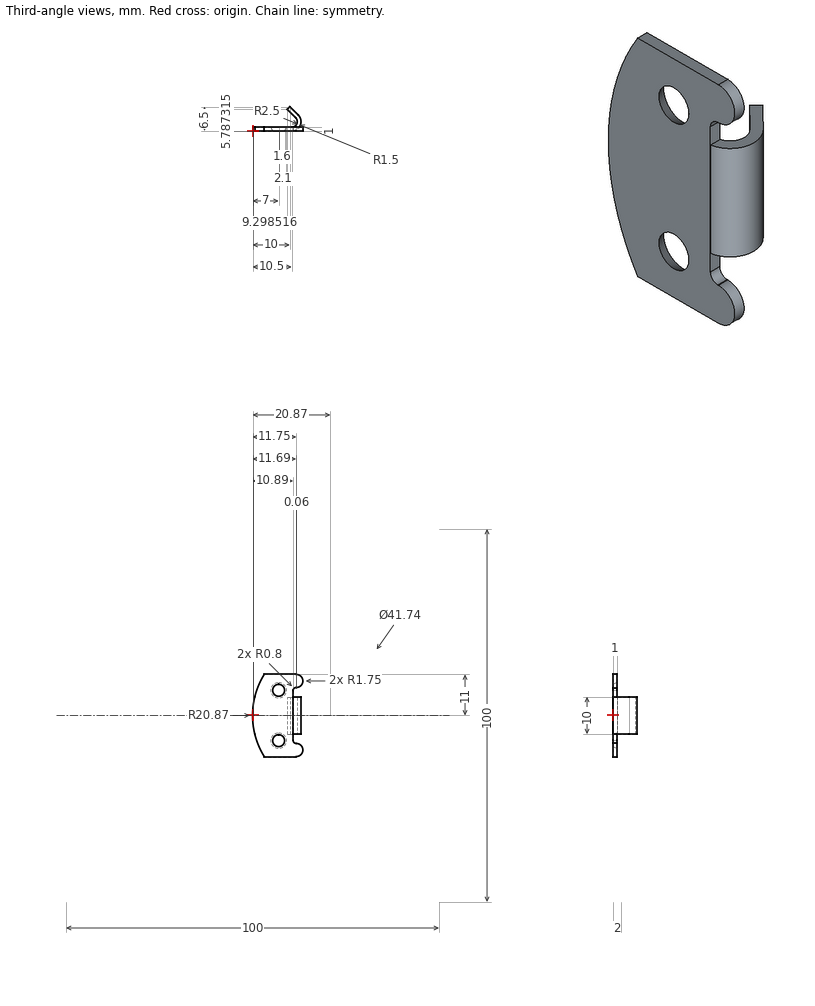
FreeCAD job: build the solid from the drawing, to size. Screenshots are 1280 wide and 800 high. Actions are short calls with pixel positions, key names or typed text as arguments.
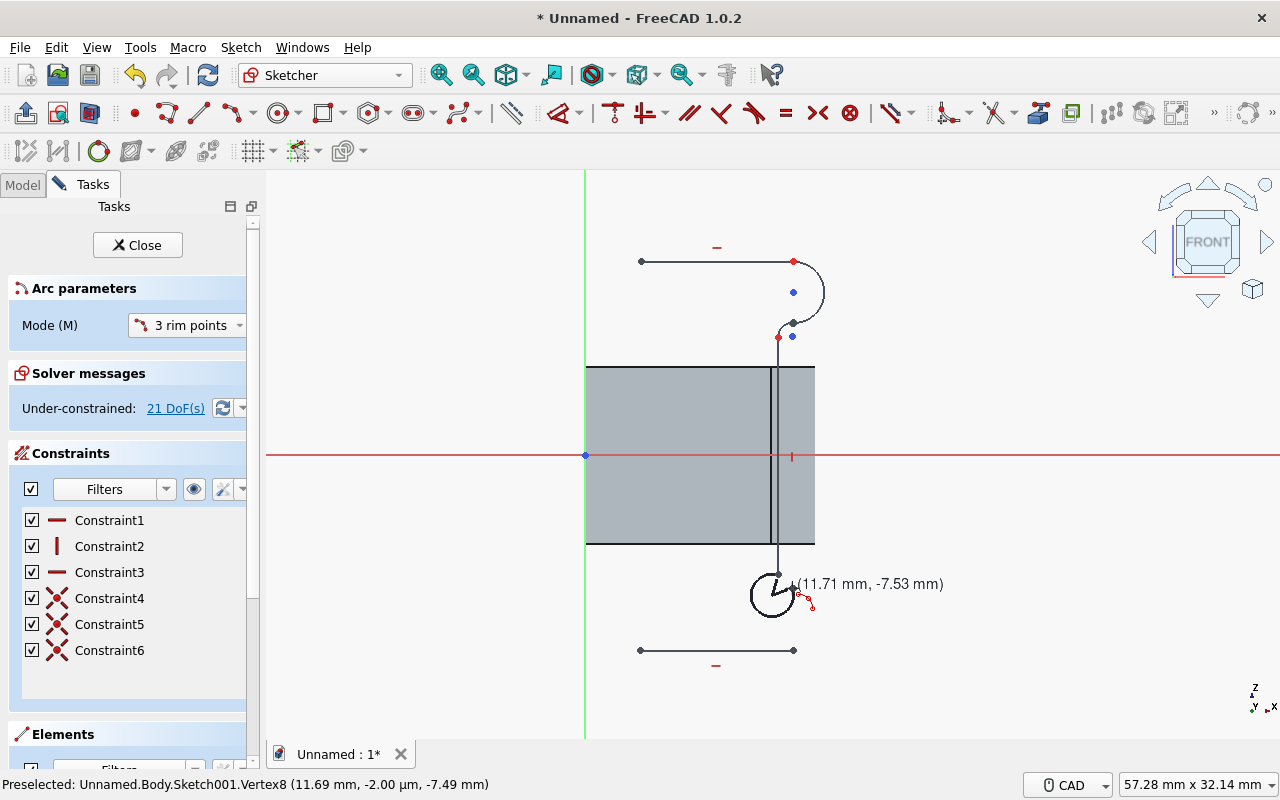
scroll(782, 584, up, 7)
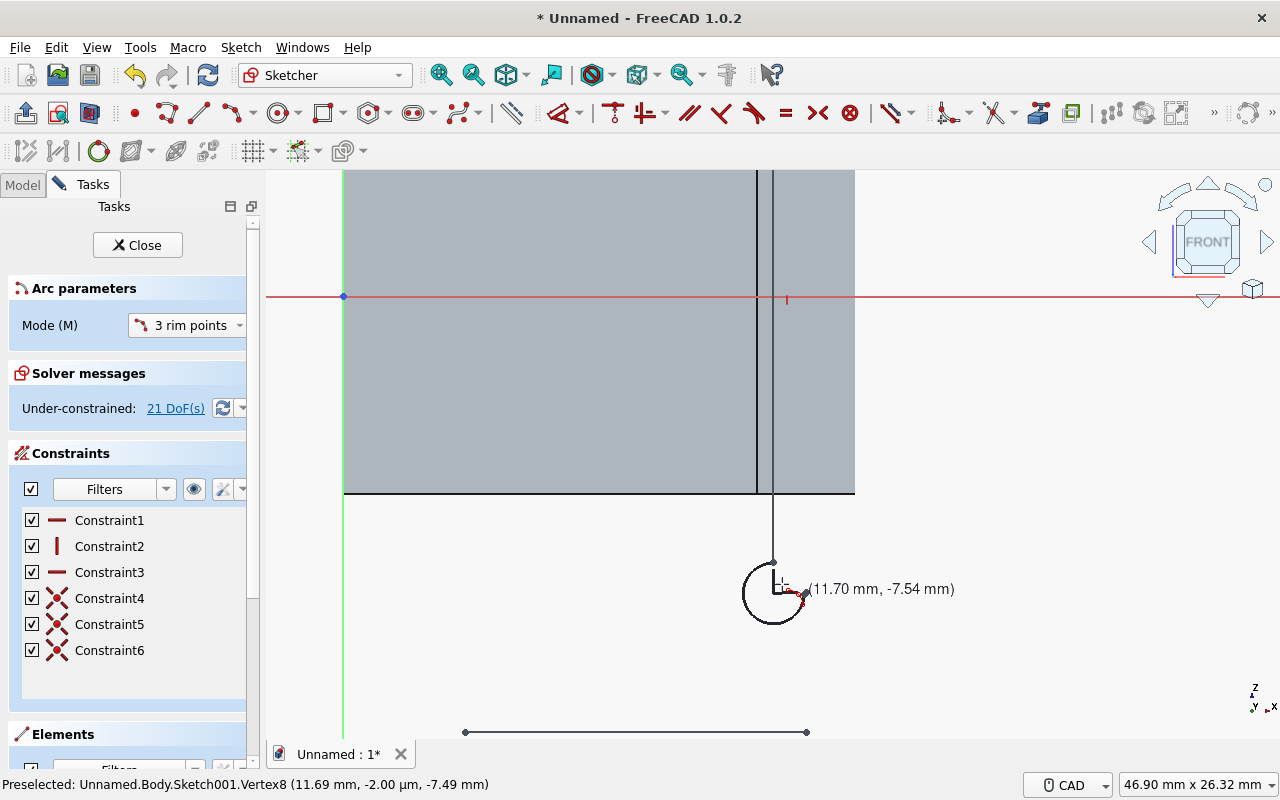
click(781, 582)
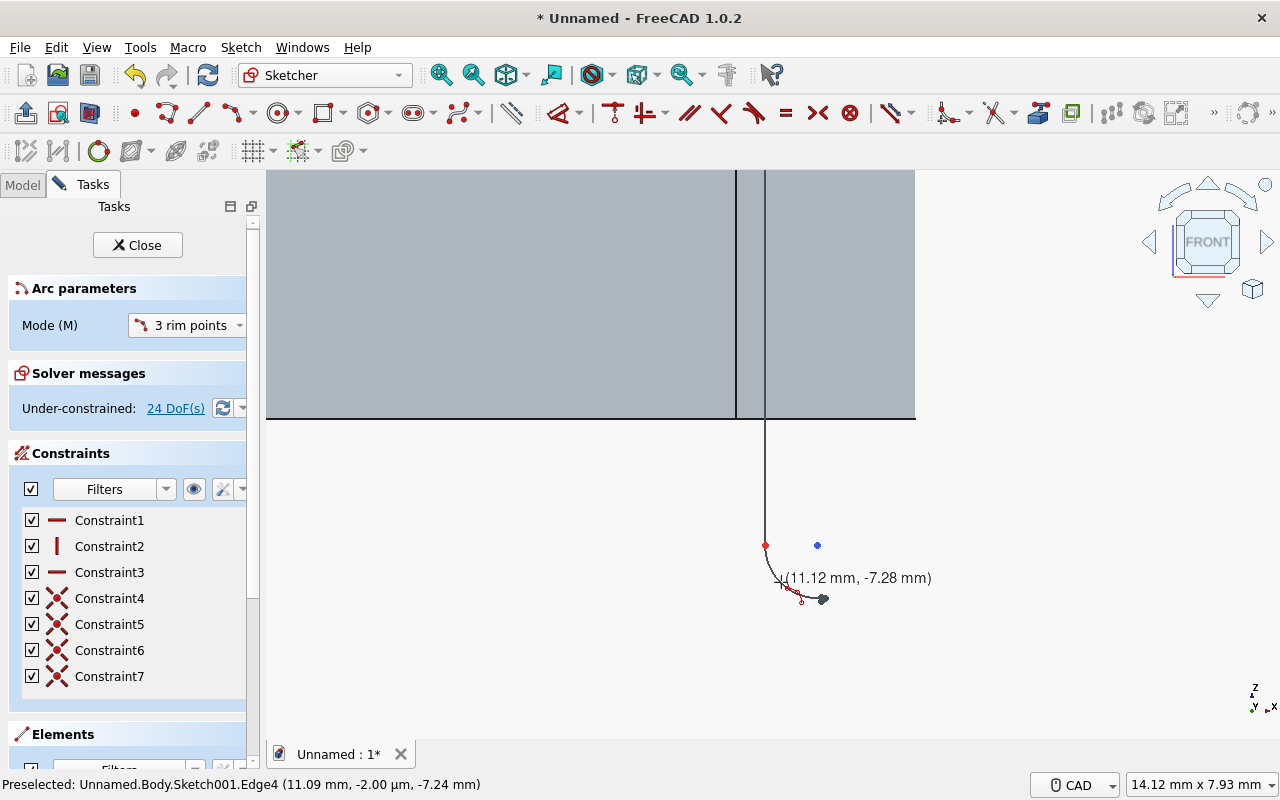
scroll(826, 599, up, 10)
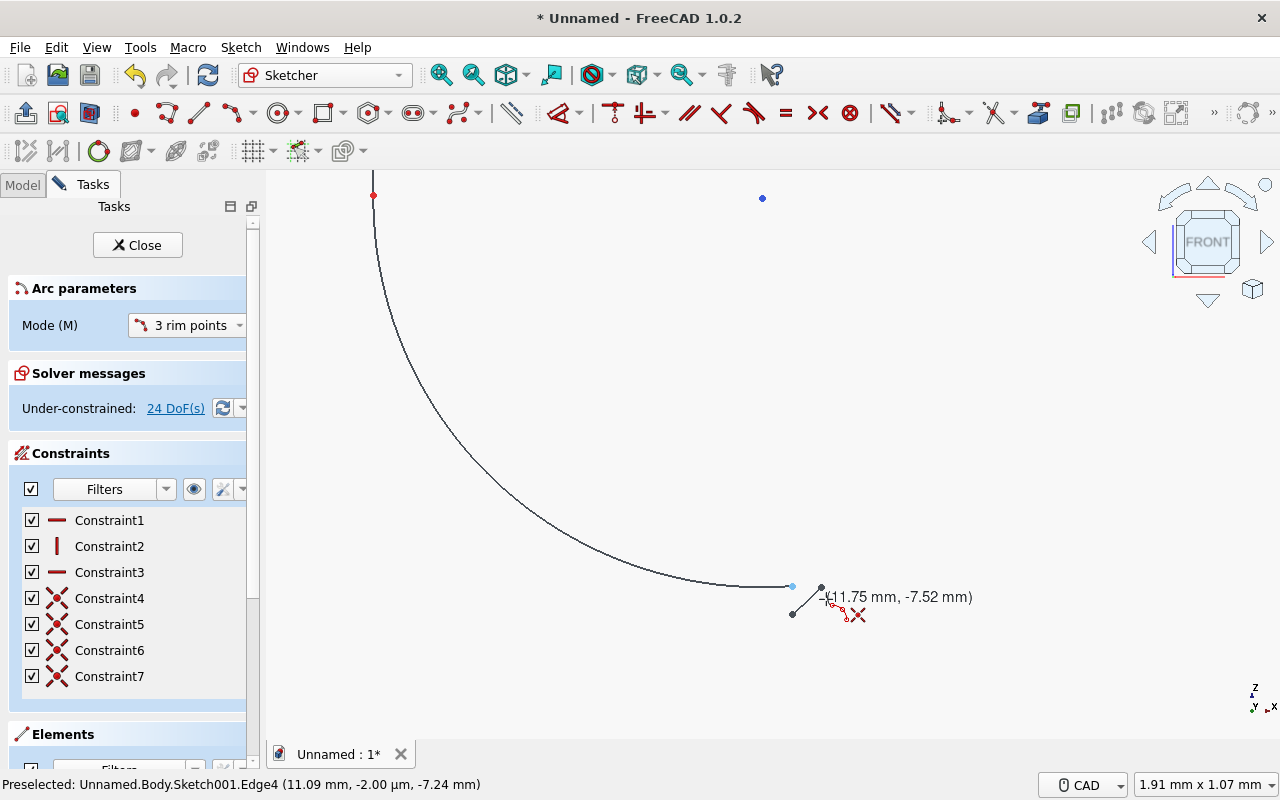
click(821, 587)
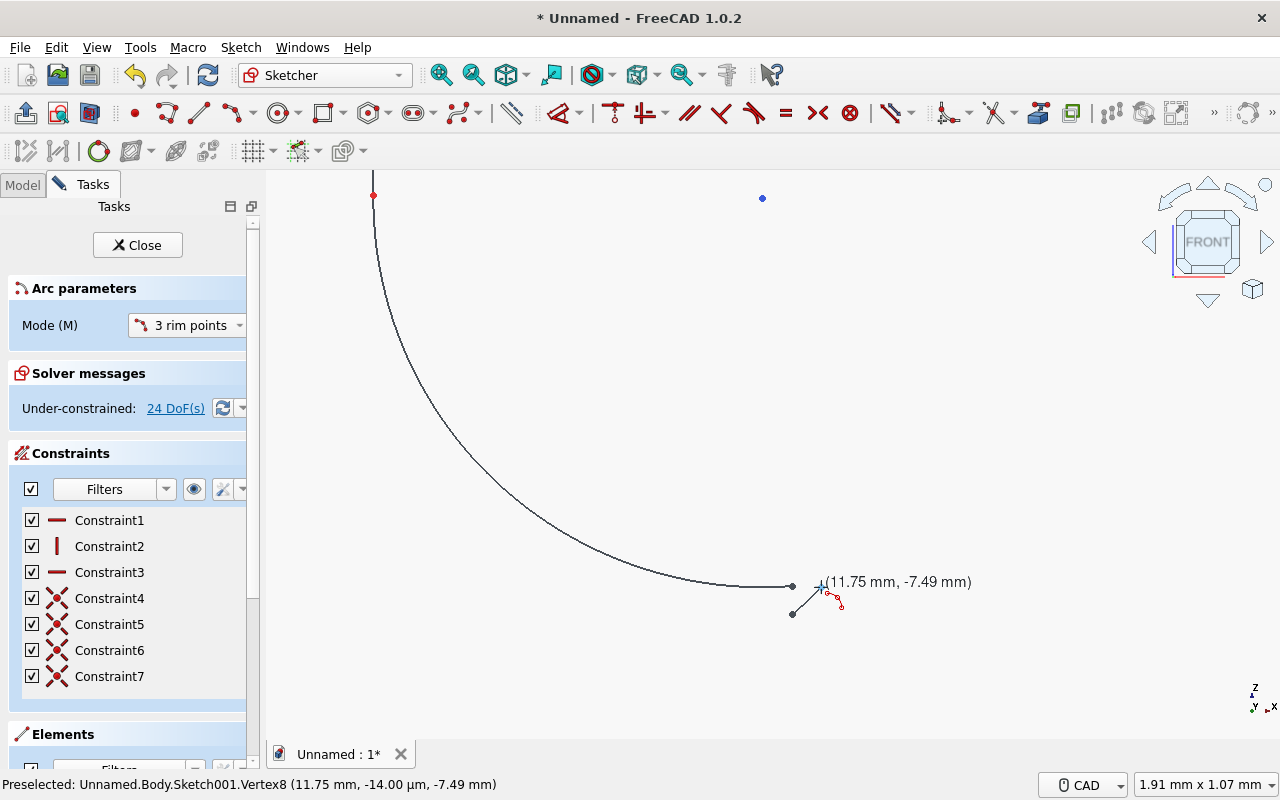
scroll(792, 587, down, 17)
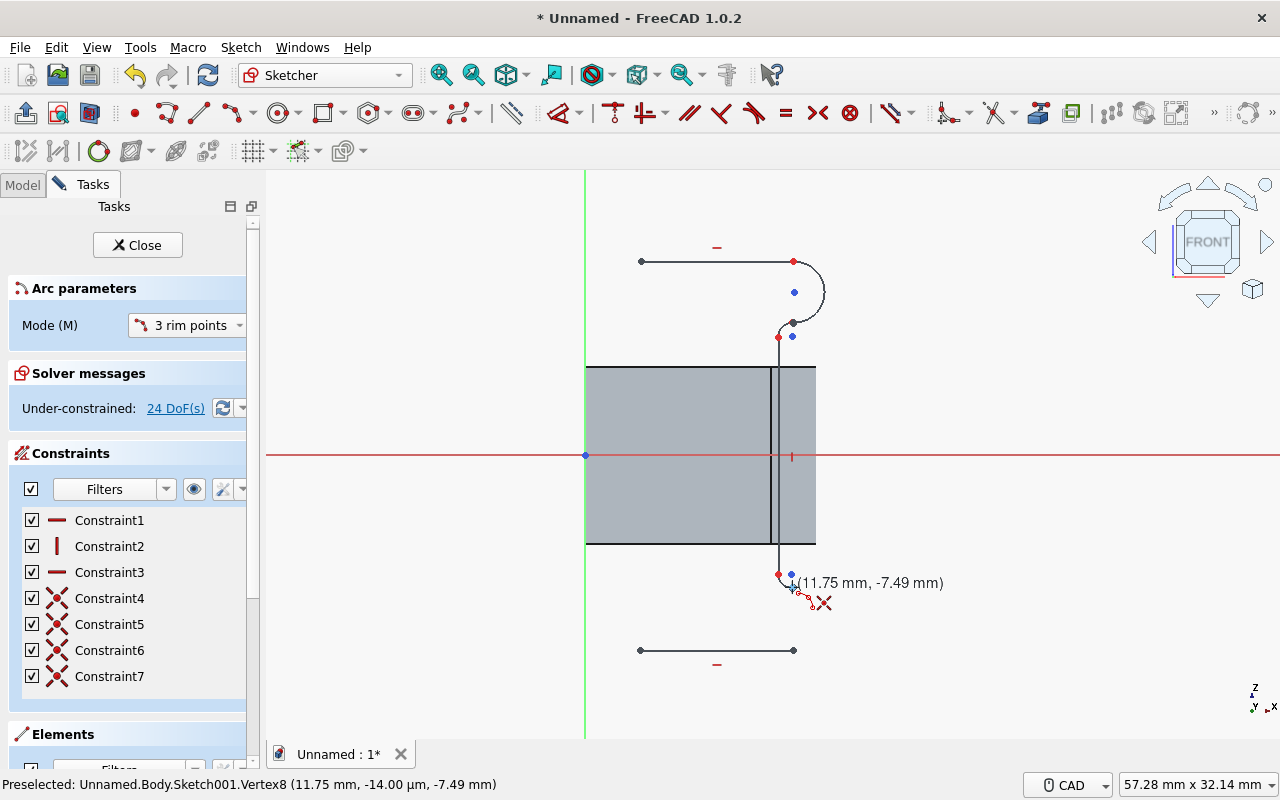
click(794, 651)
click(824, 619)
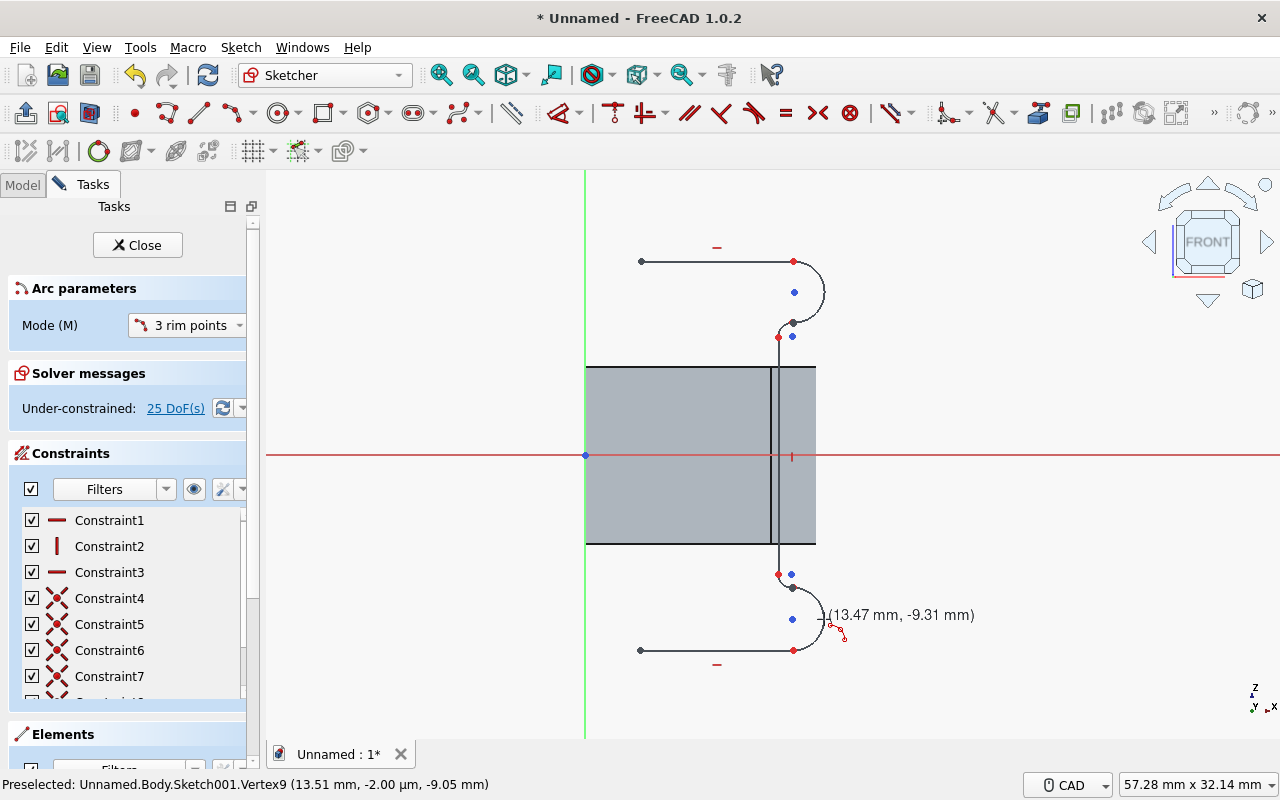
click(641, 651)
click(641, 262)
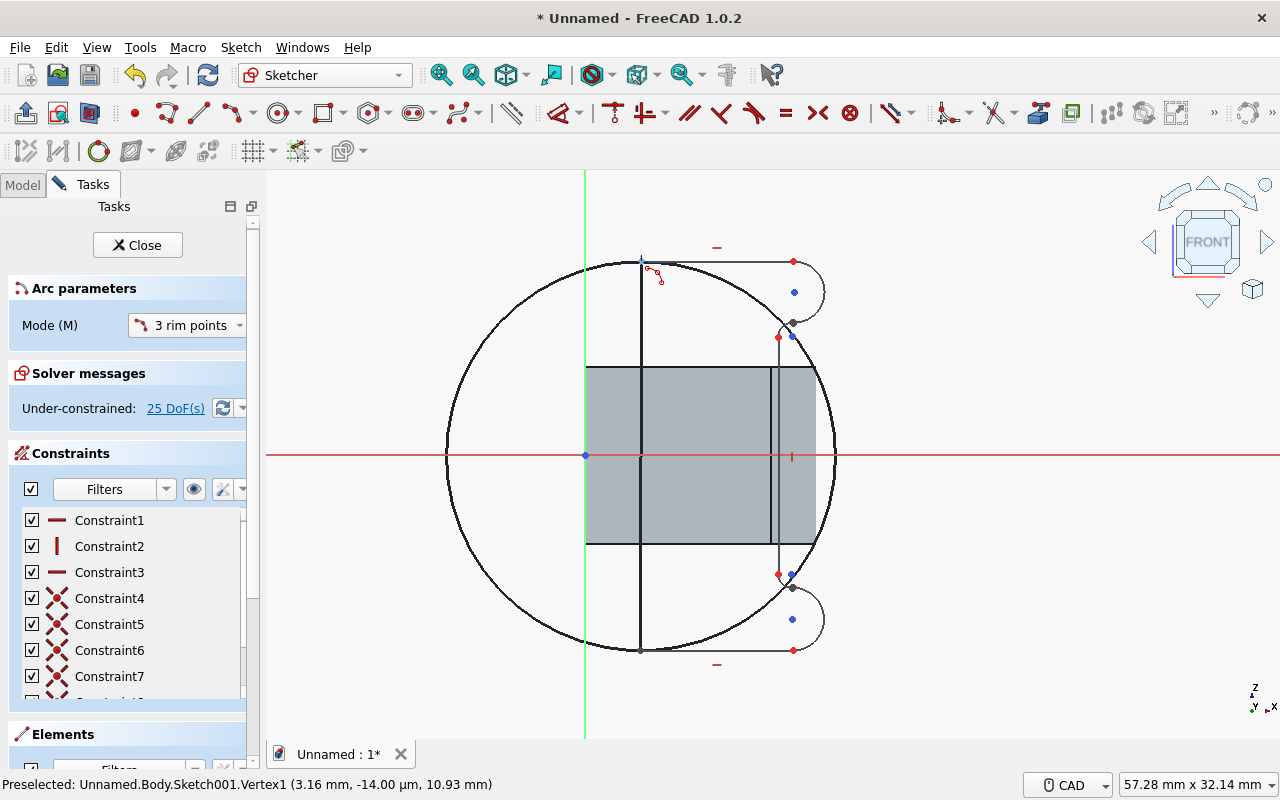
scroll(595, 374, up, 3)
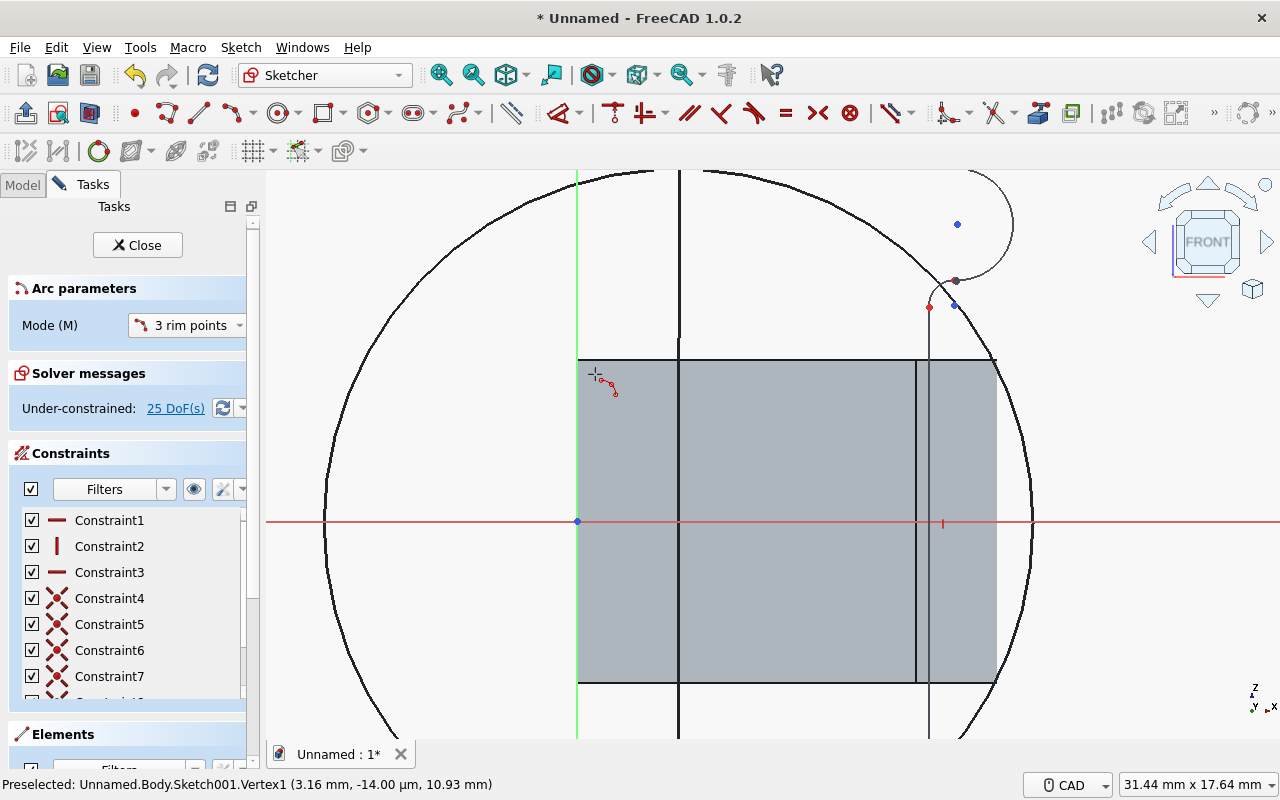
click(594, 373)
key(Escape)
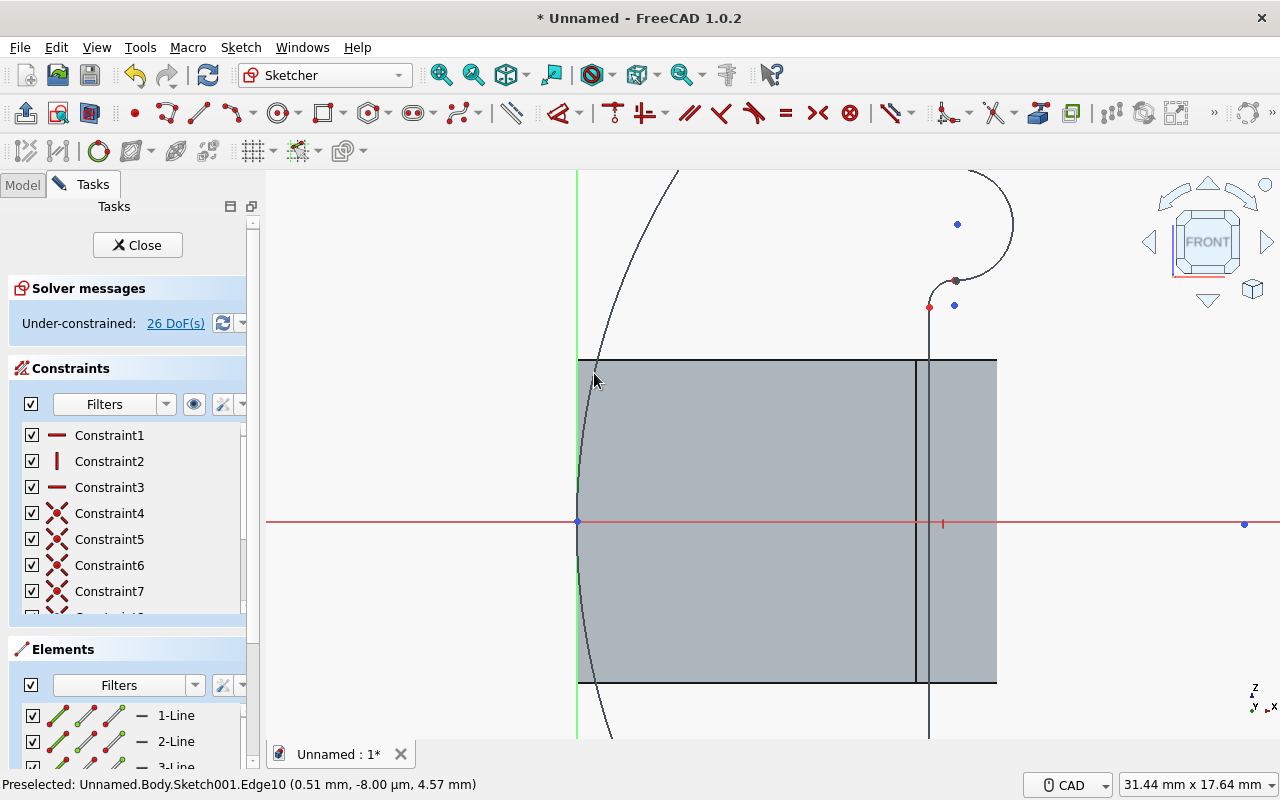
scroll(594, 373, down, 3)